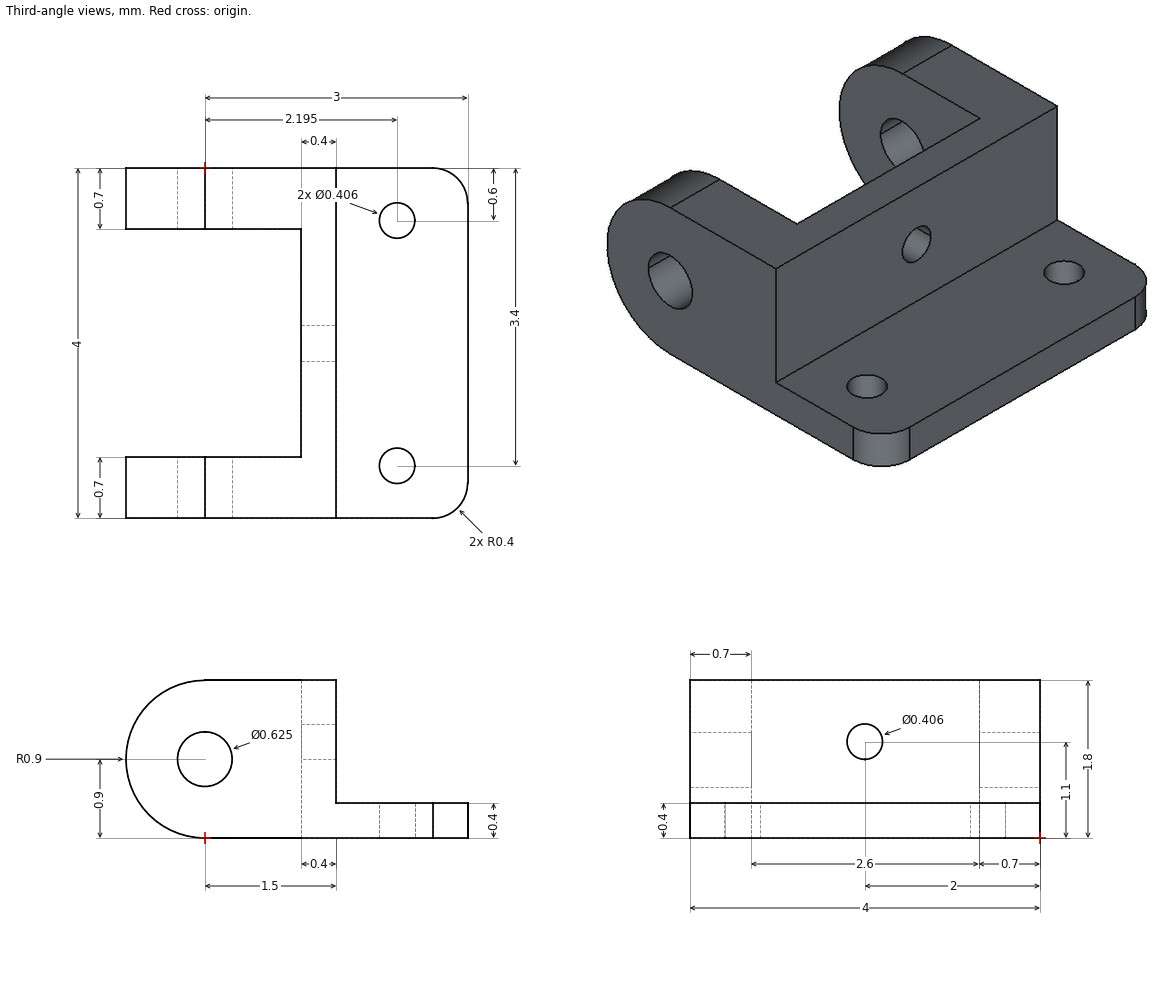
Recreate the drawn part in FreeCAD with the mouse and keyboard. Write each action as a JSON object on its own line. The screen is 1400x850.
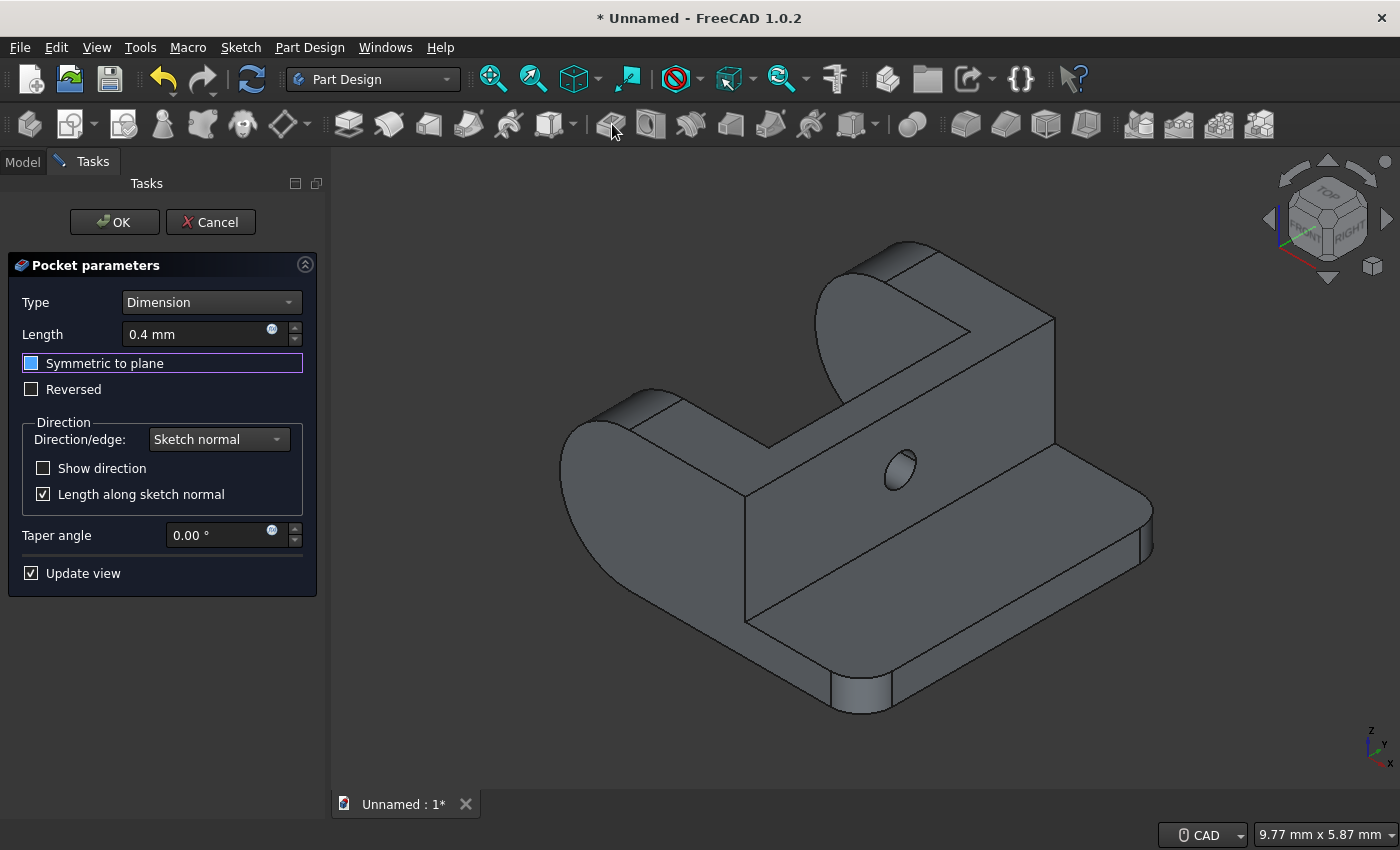
{"action": "left_click", "coordinate": [115, 222]}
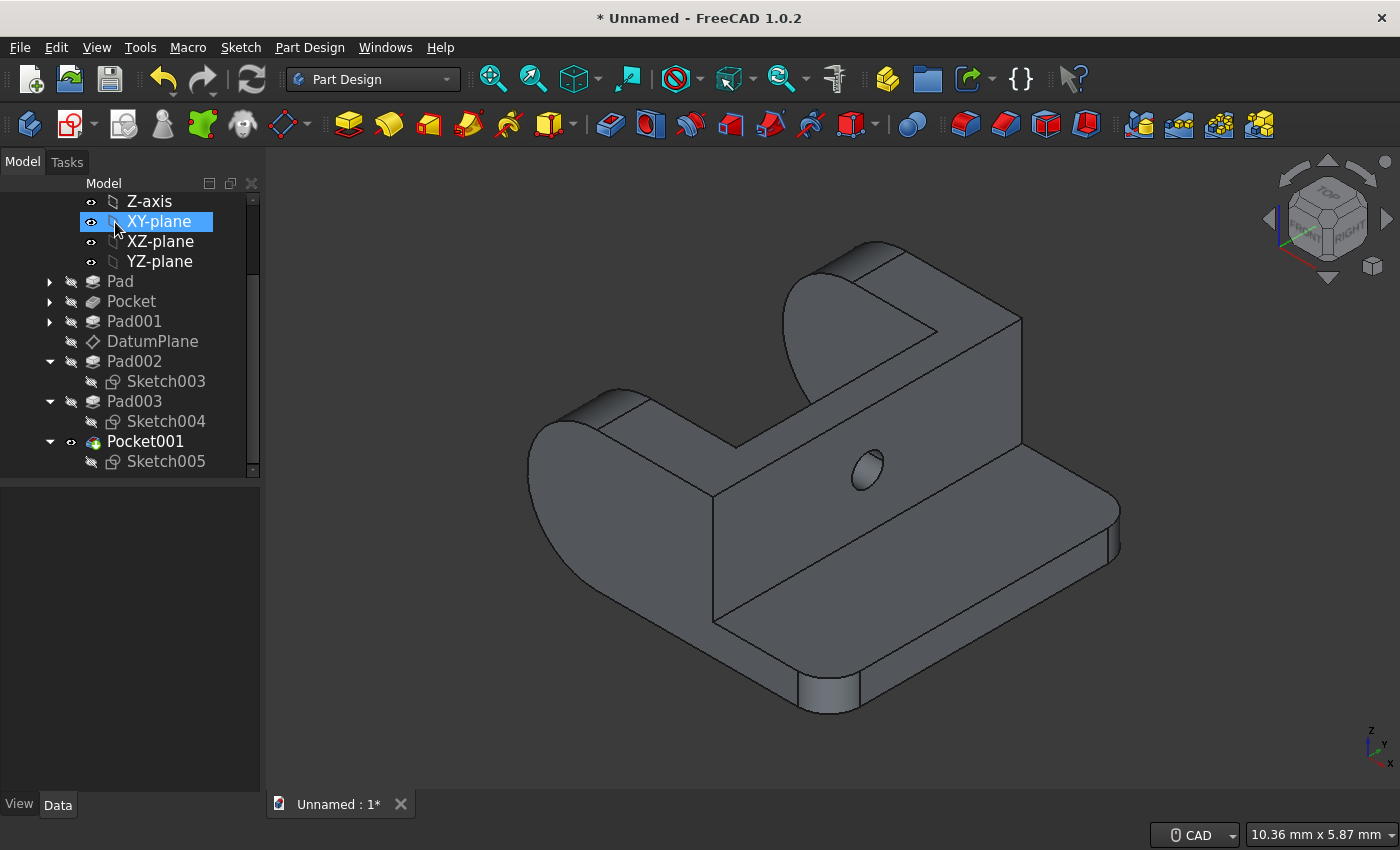
{"action": "left_click", "coordinate": [1014, 514]}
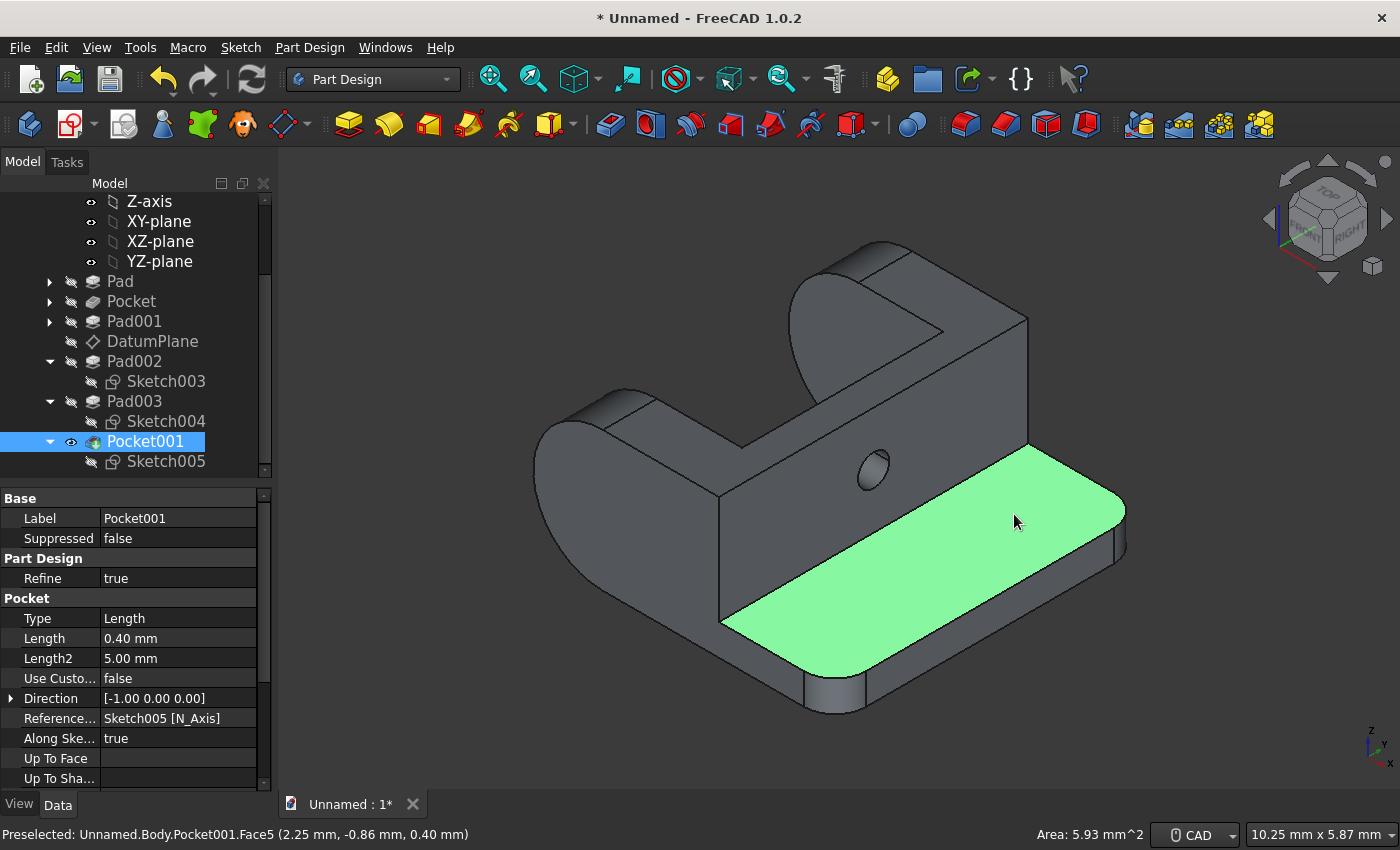
{"action": "left_click", "coordinate": [70, 124]}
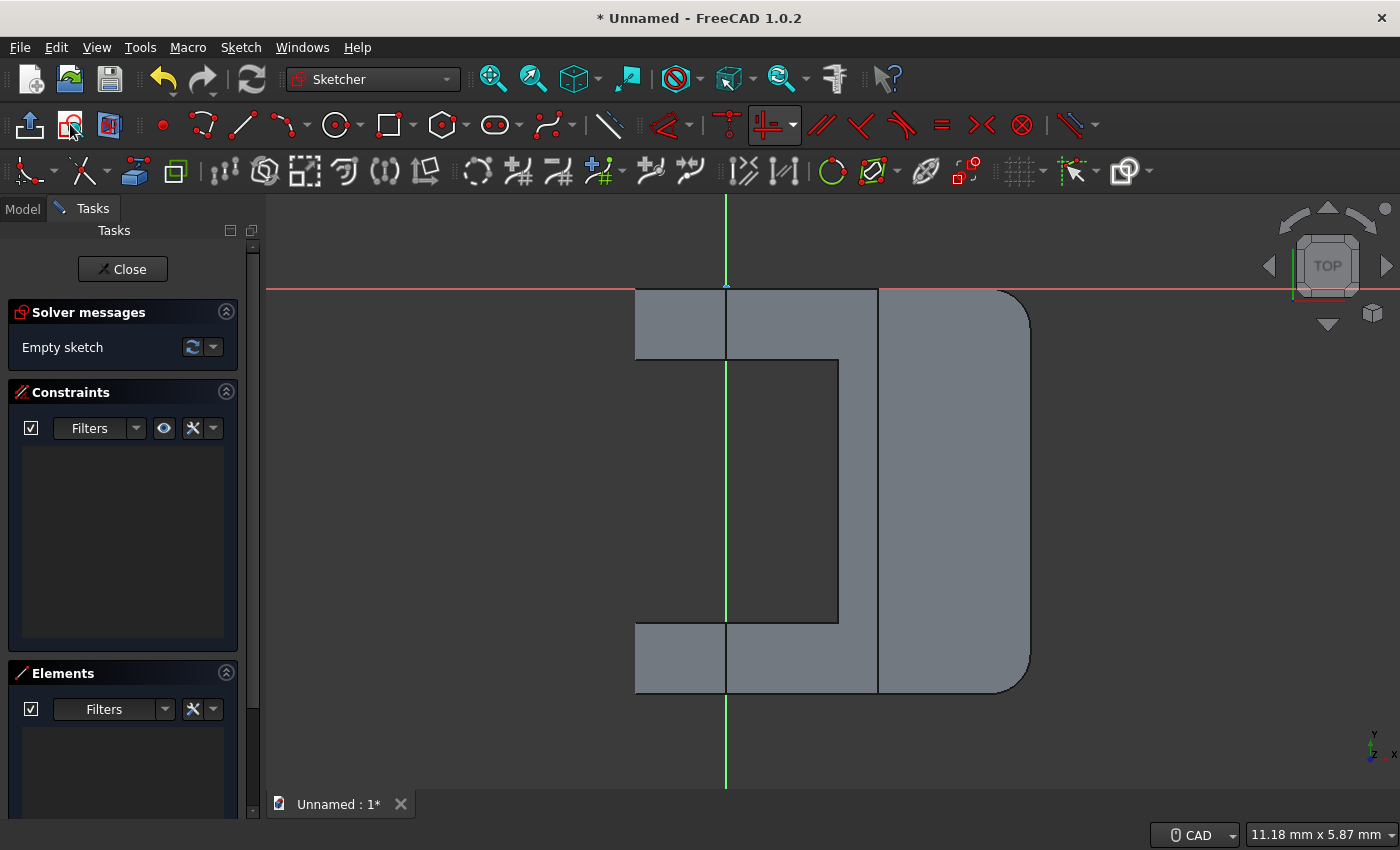
{"action": "key", "text": "q s"}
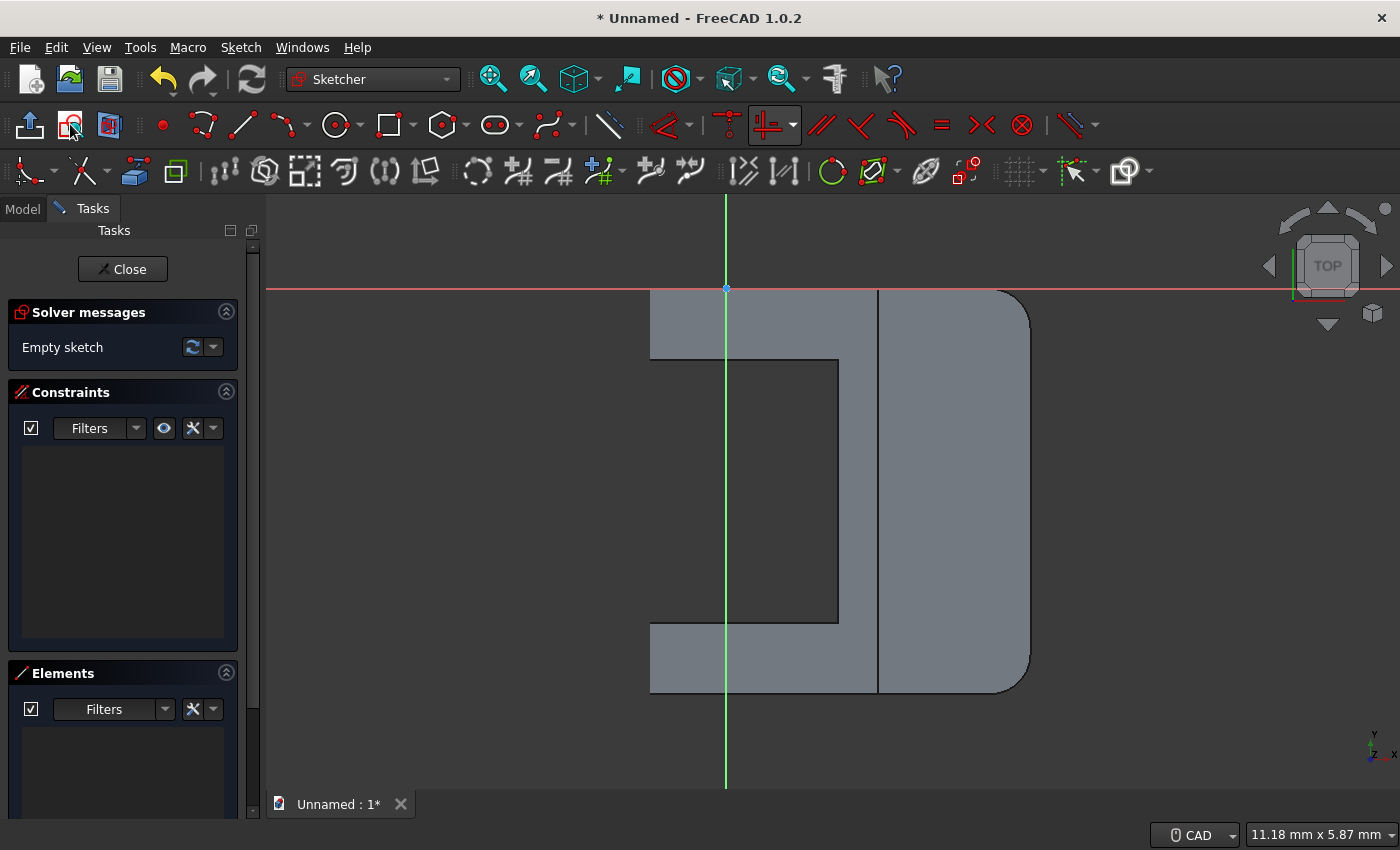
{"action": "key", "text": "g c"}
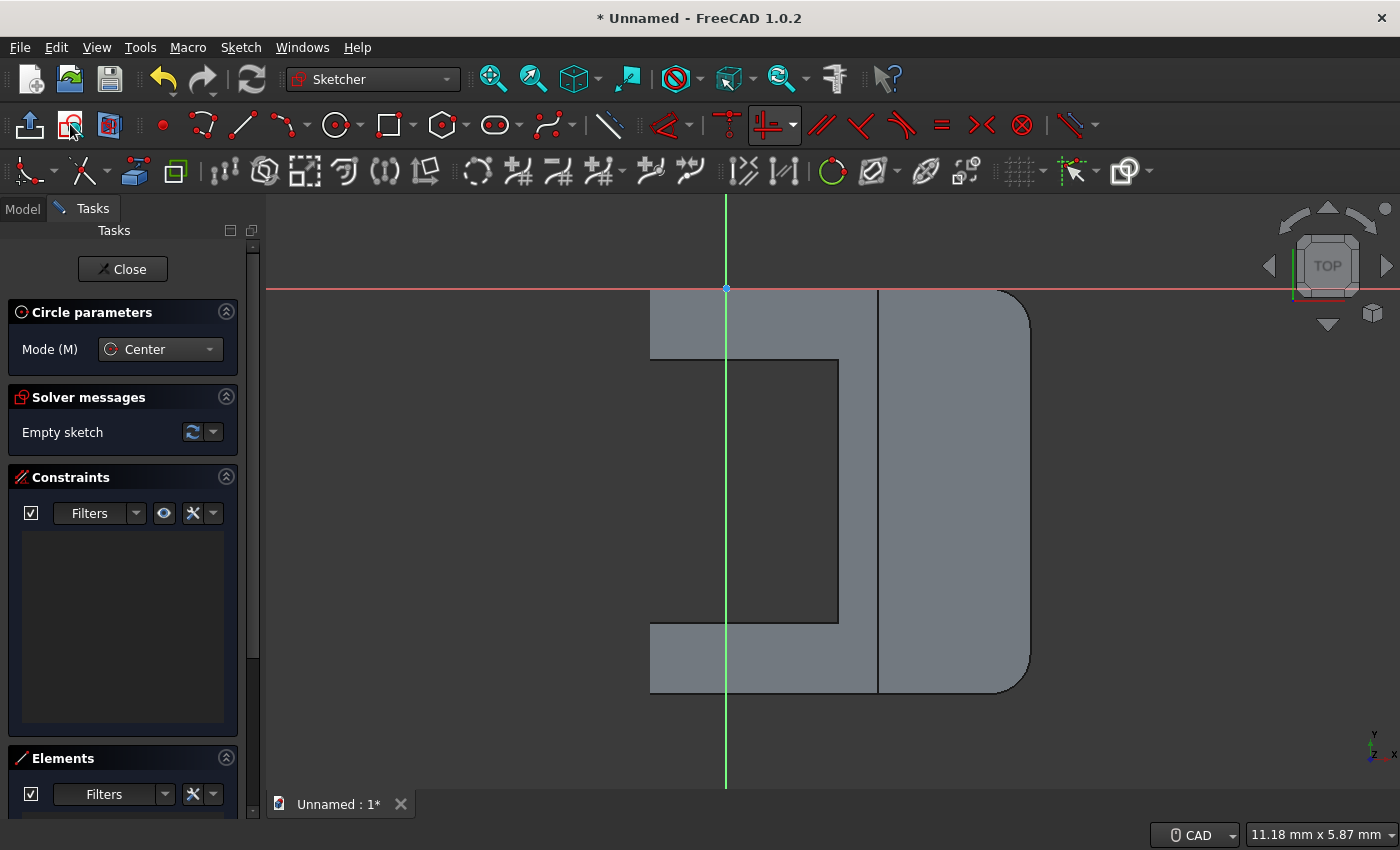
{"action": "left_click", "coordinate": [949, 350]}
{"action": "mouse_move", "coordinate": [964, 335]}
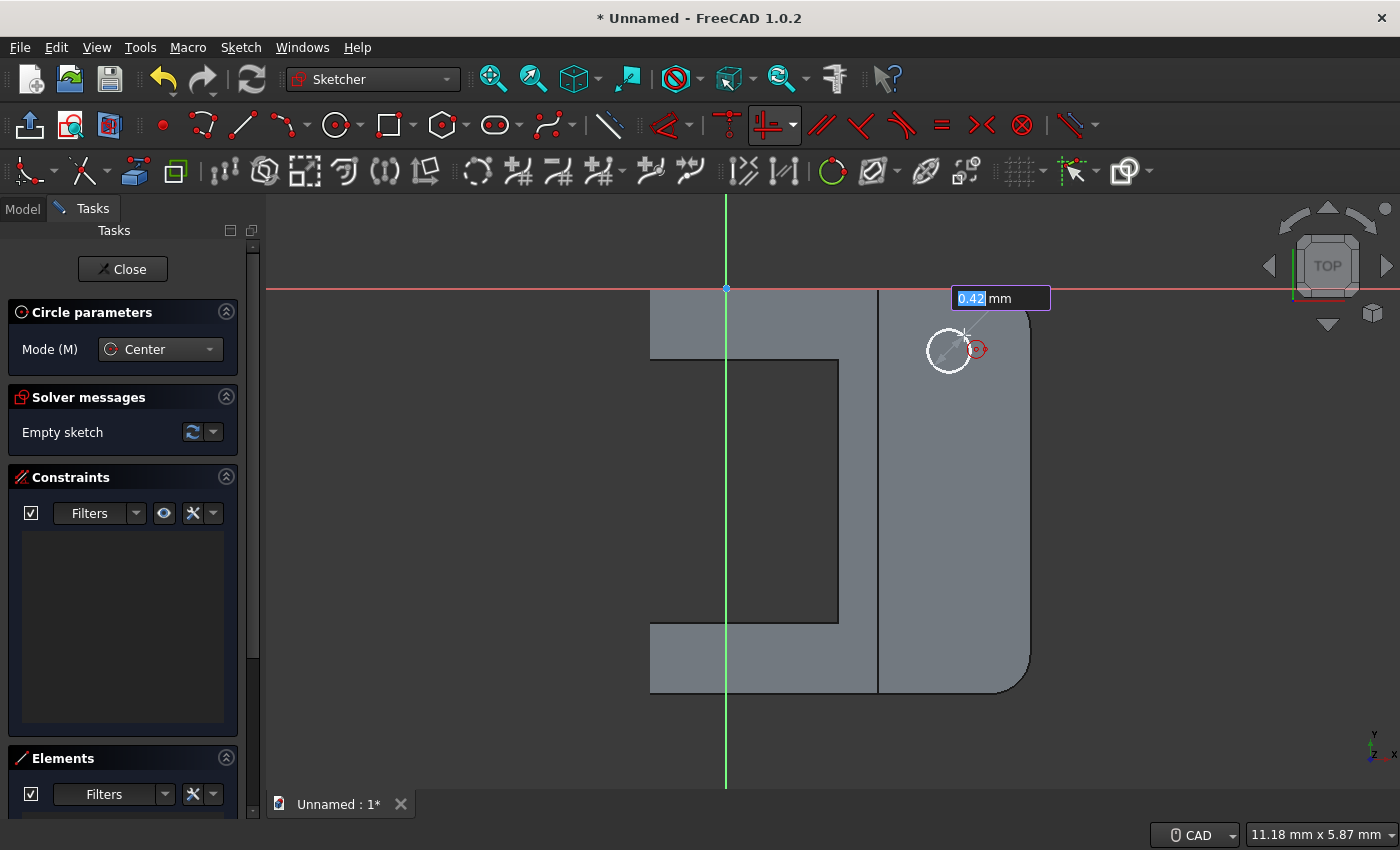
{"action": "type", "text": "0.406"}
{"action": "key", "text": "Return"}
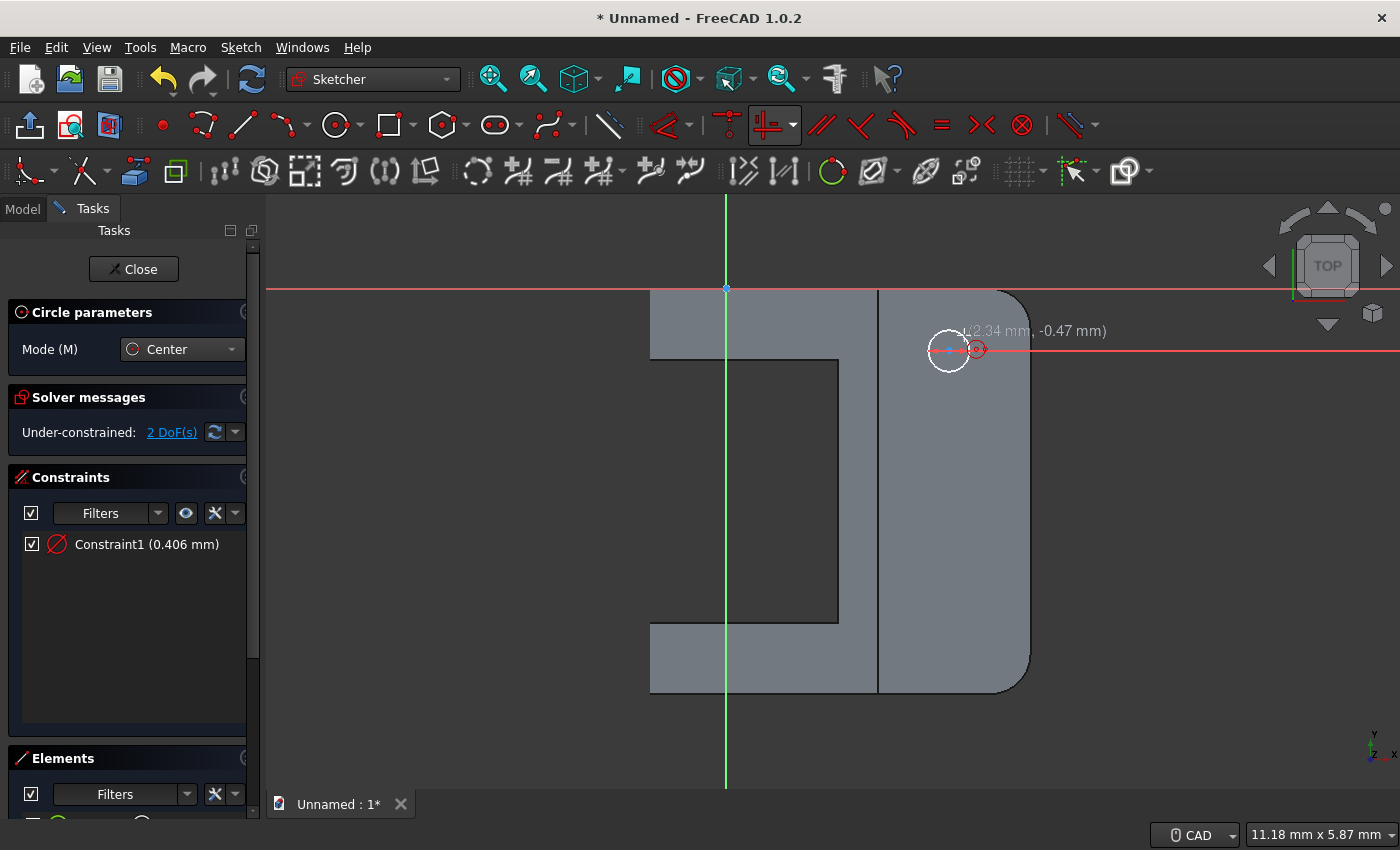
{"action": "left_click", "coordinate": [949, 633]}
{"action": "mouse_move", "coordinate": [964, 619]}